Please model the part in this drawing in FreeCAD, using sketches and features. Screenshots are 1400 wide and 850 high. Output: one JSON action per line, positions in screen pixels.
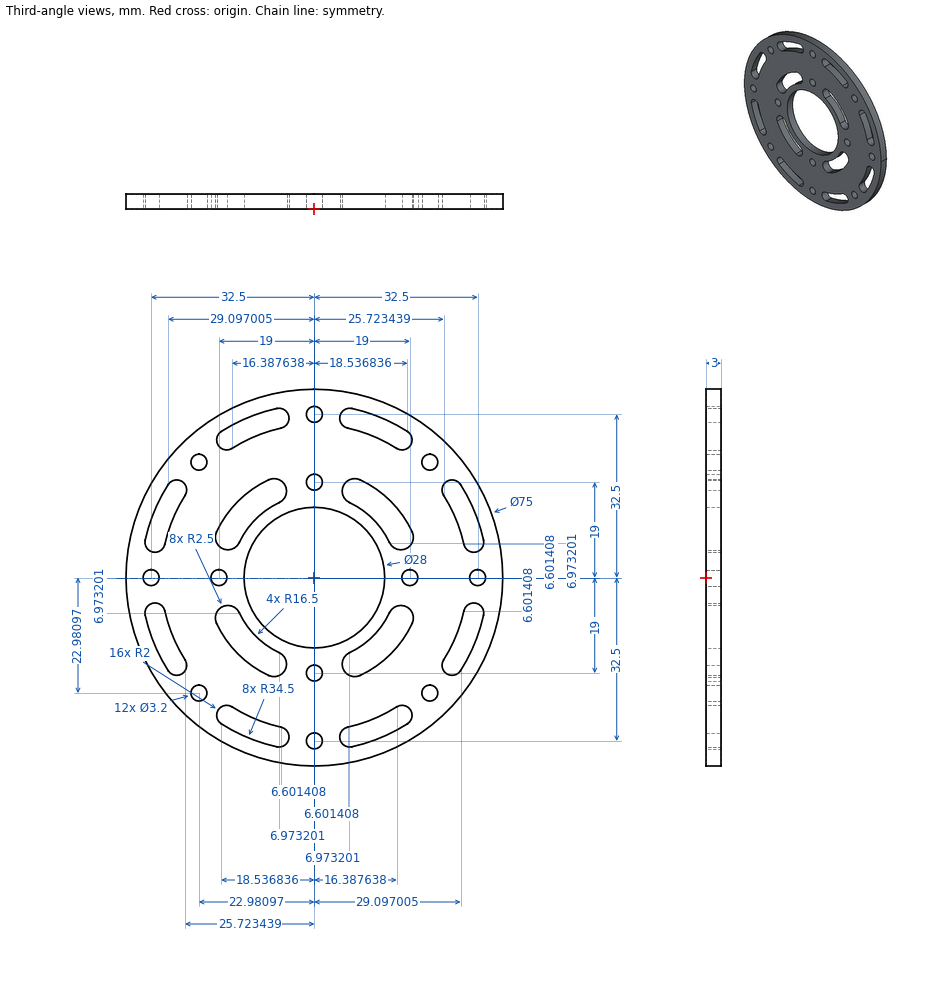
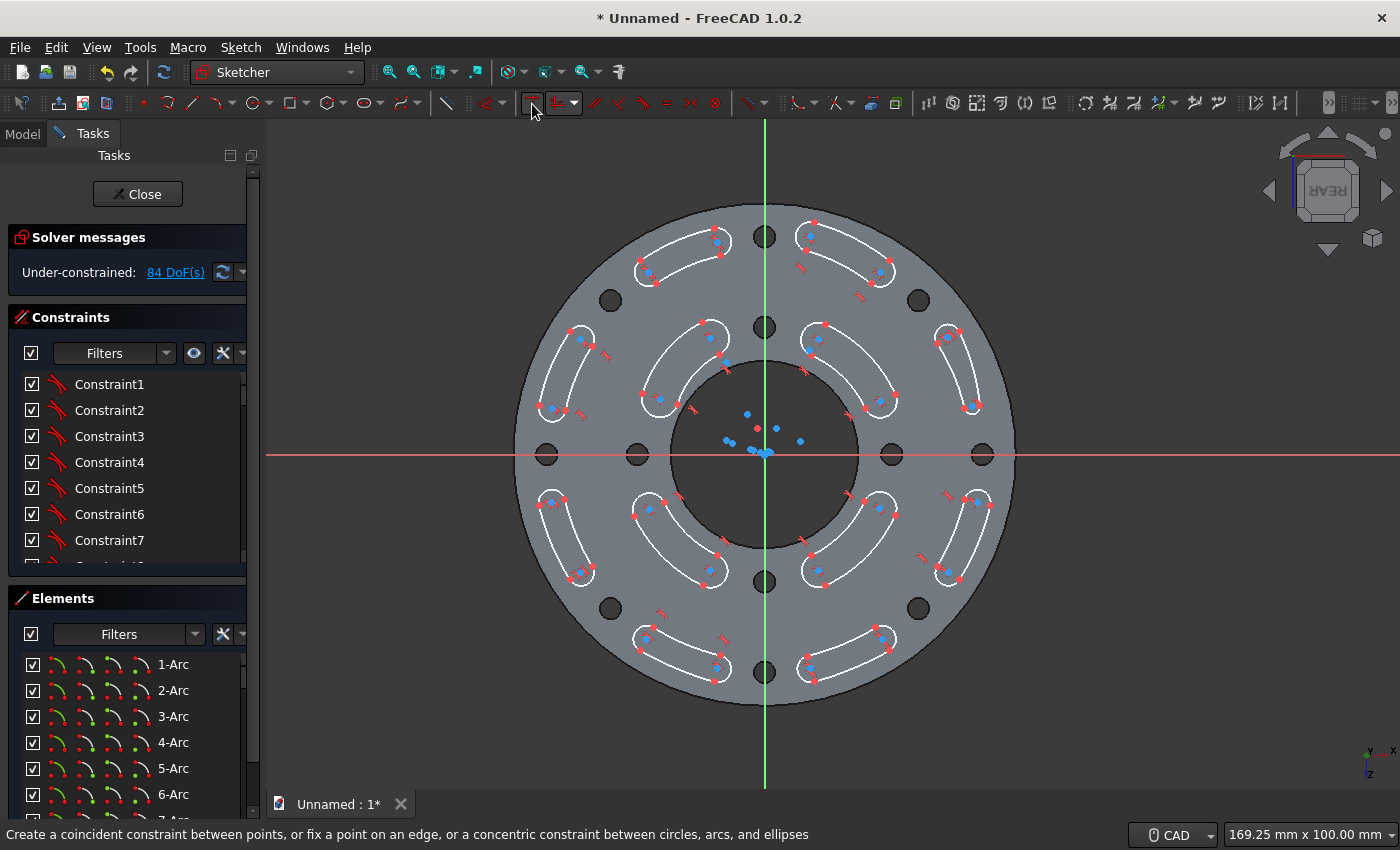
{"action": "left_click", "coordinate": [691, 235]}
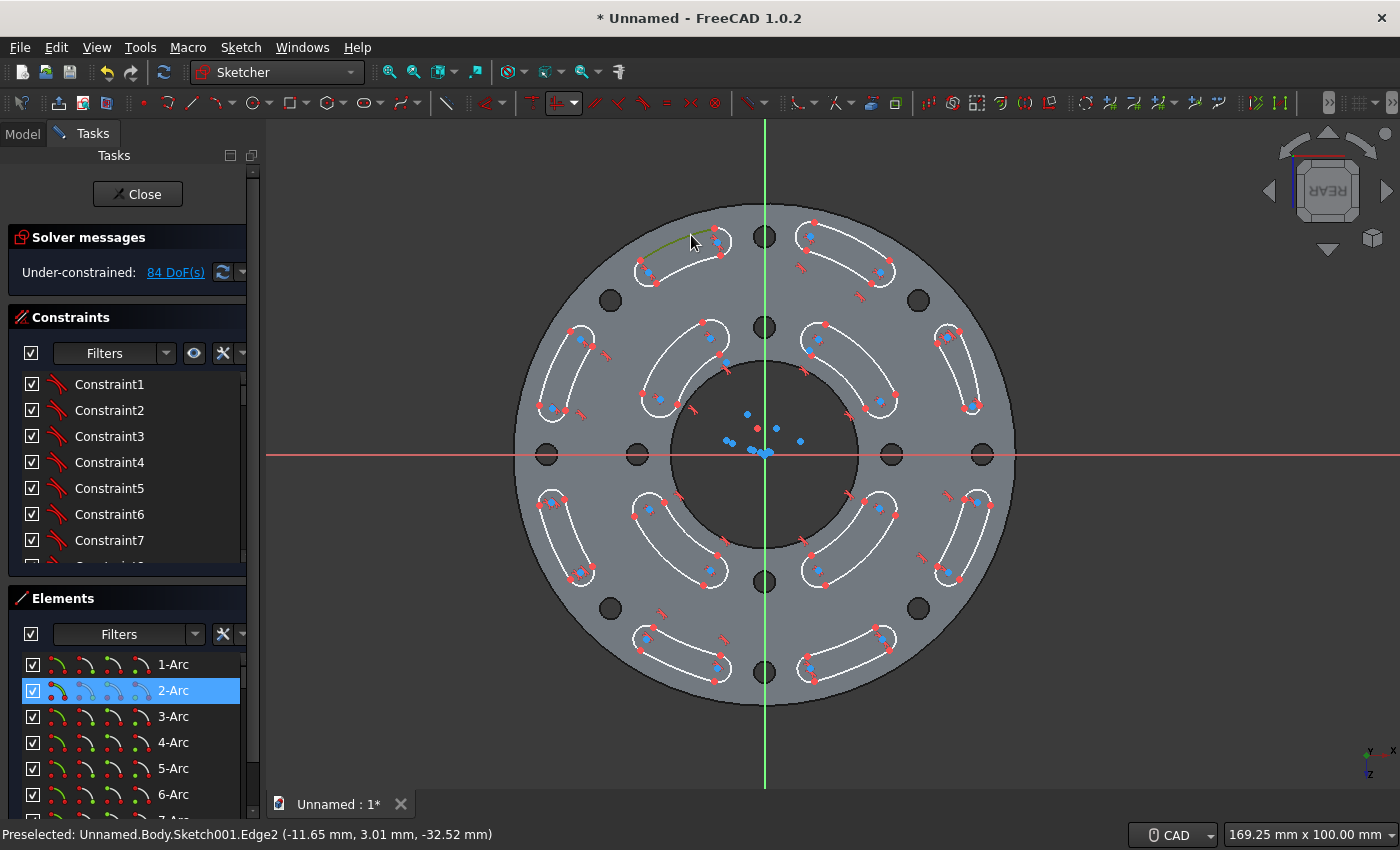
{"action": "left_click", "coordinate": [959, 388]}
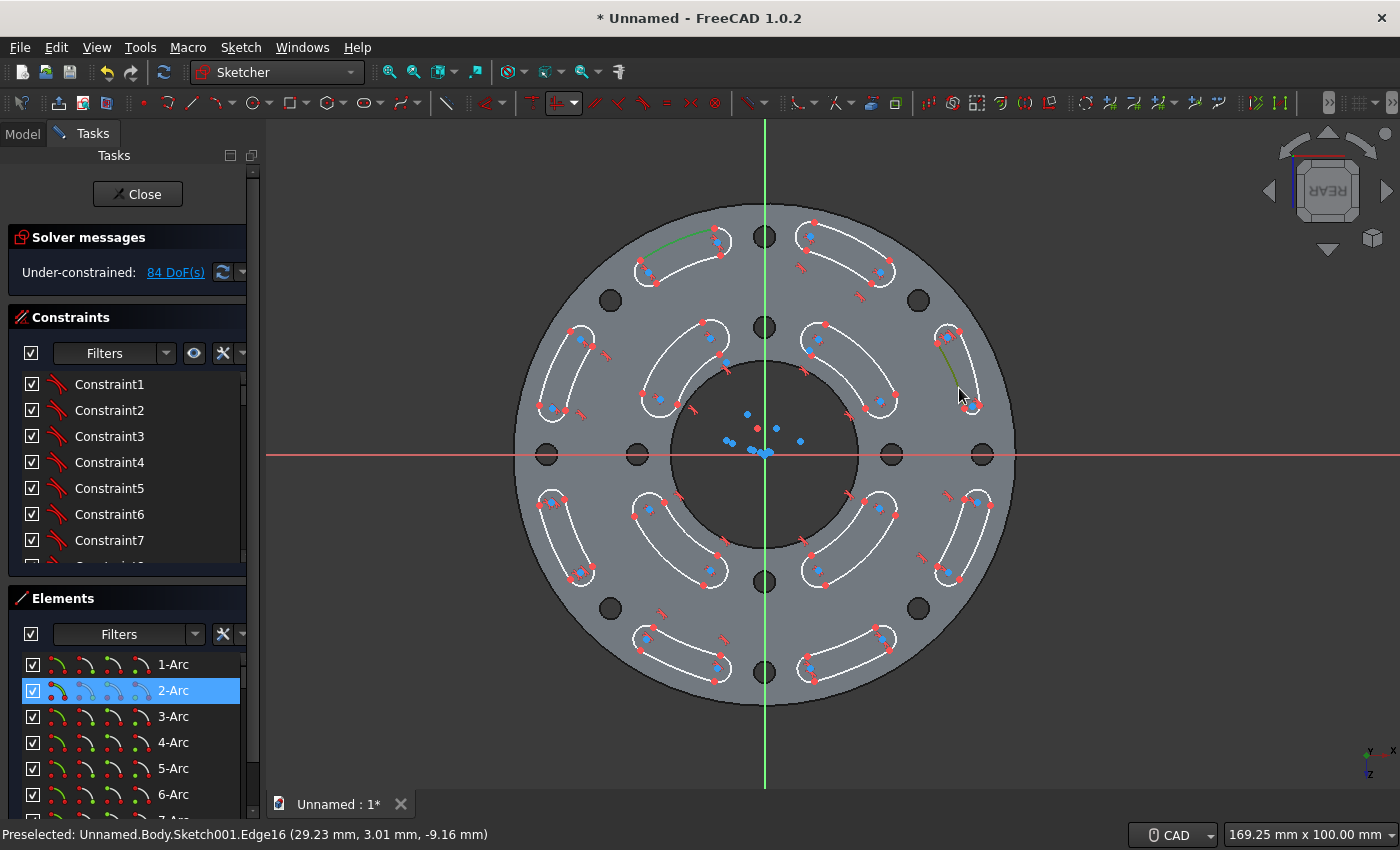
{"action": "left_click", "coordinate": [532, 104]}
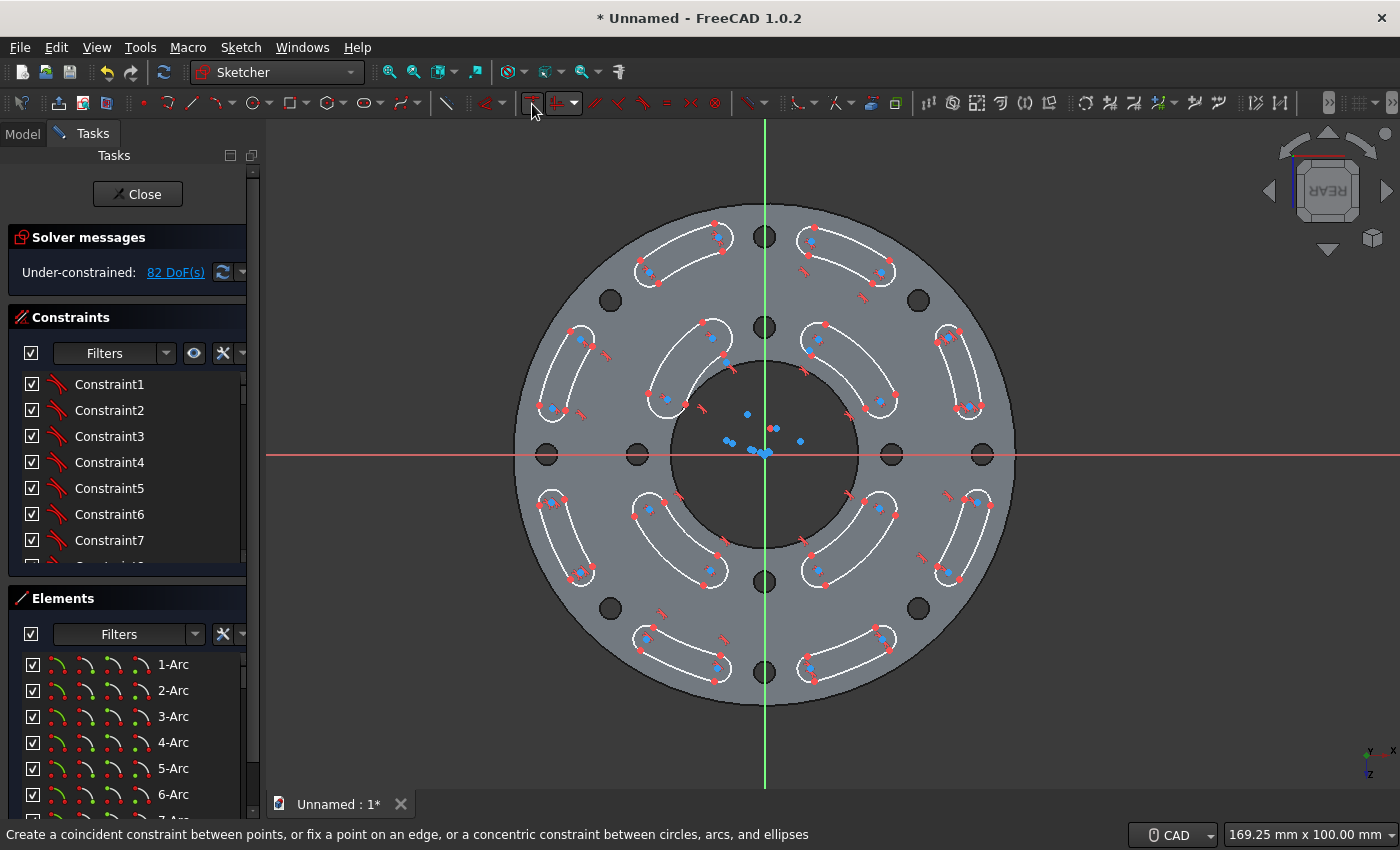
{"action": "left_click", "coordinate": [691, 232]}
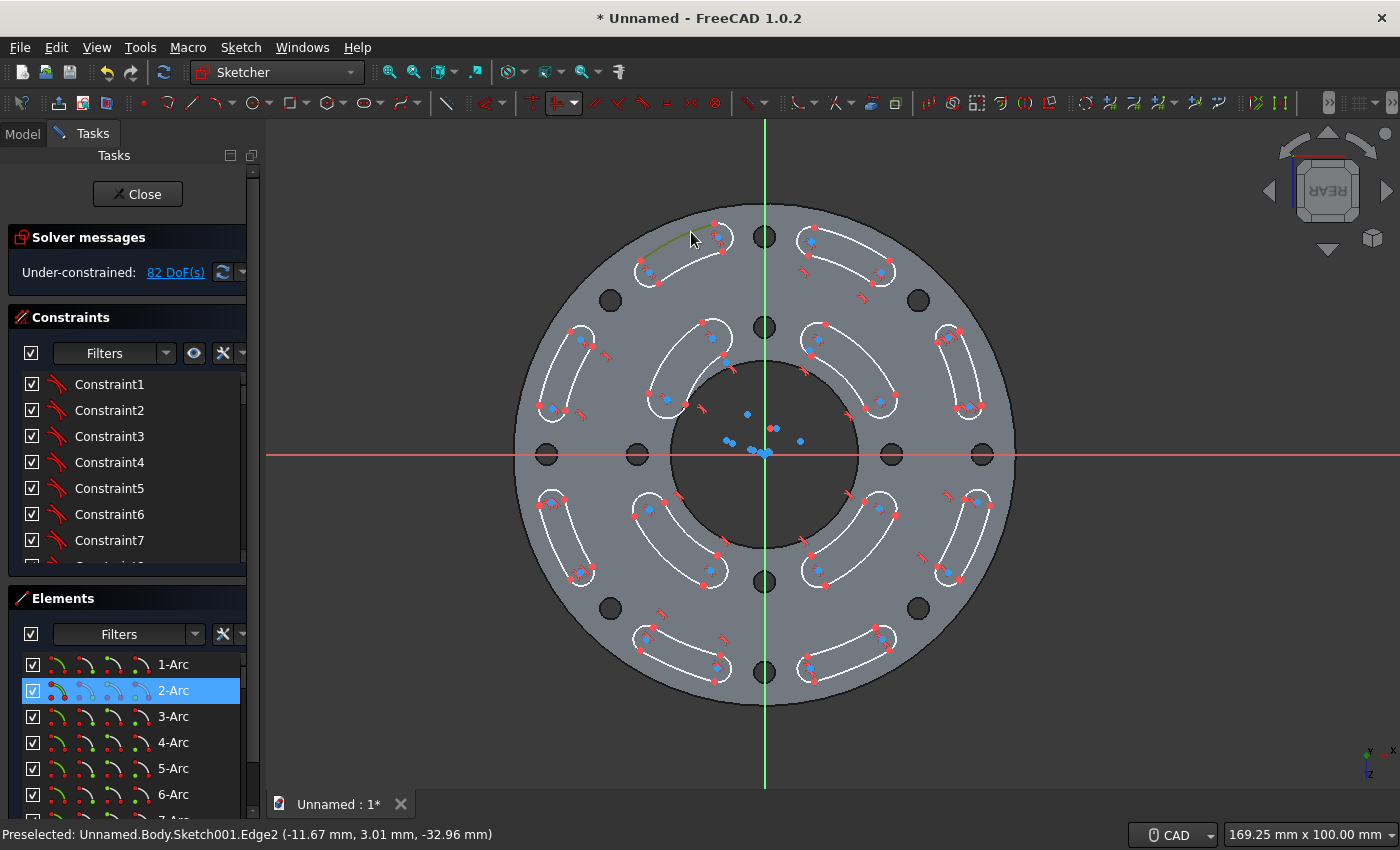
{"action": "left_click", "coordinate": [948, 547]}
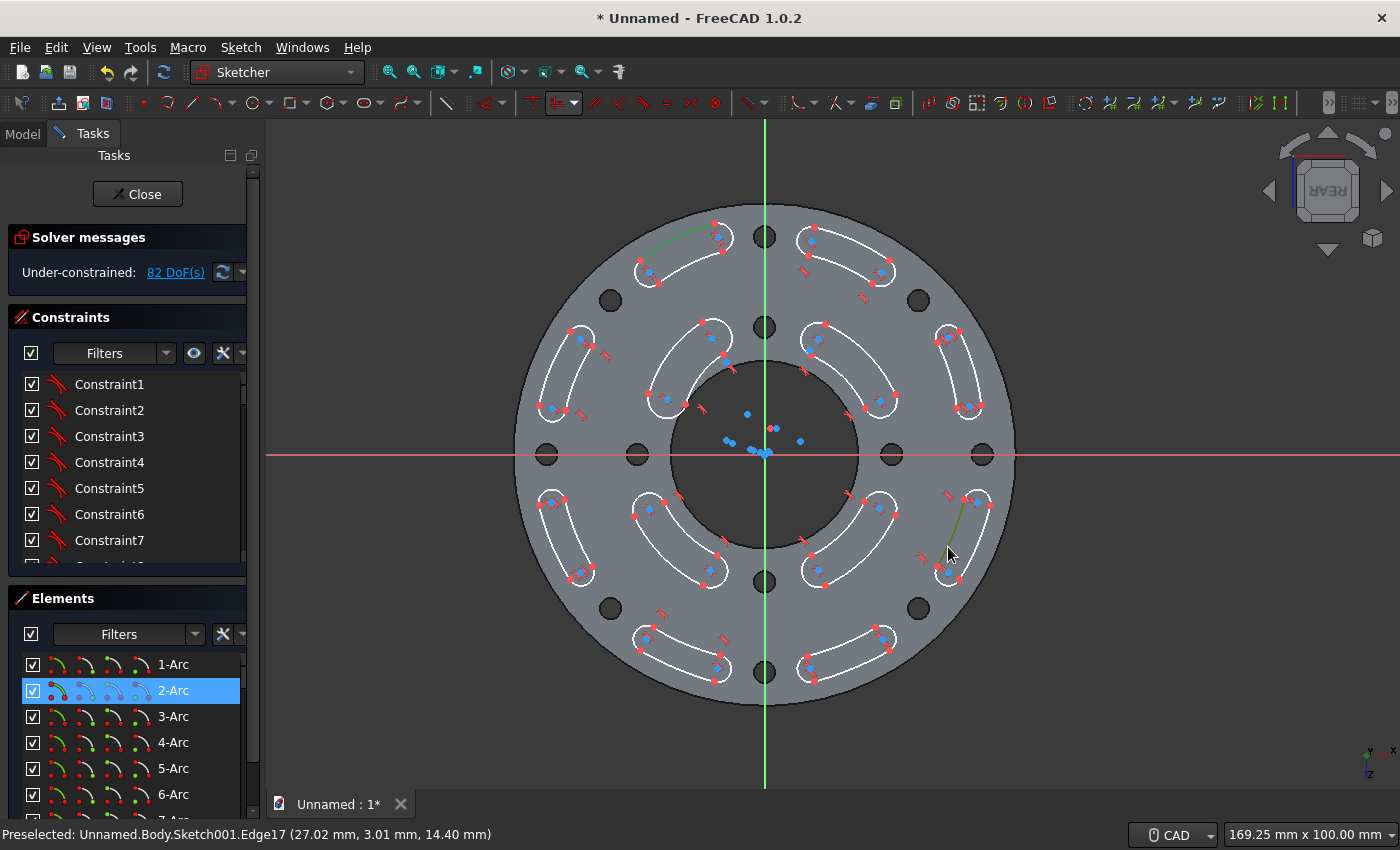
{"action": "left_click", "coordinate": [532, 104]}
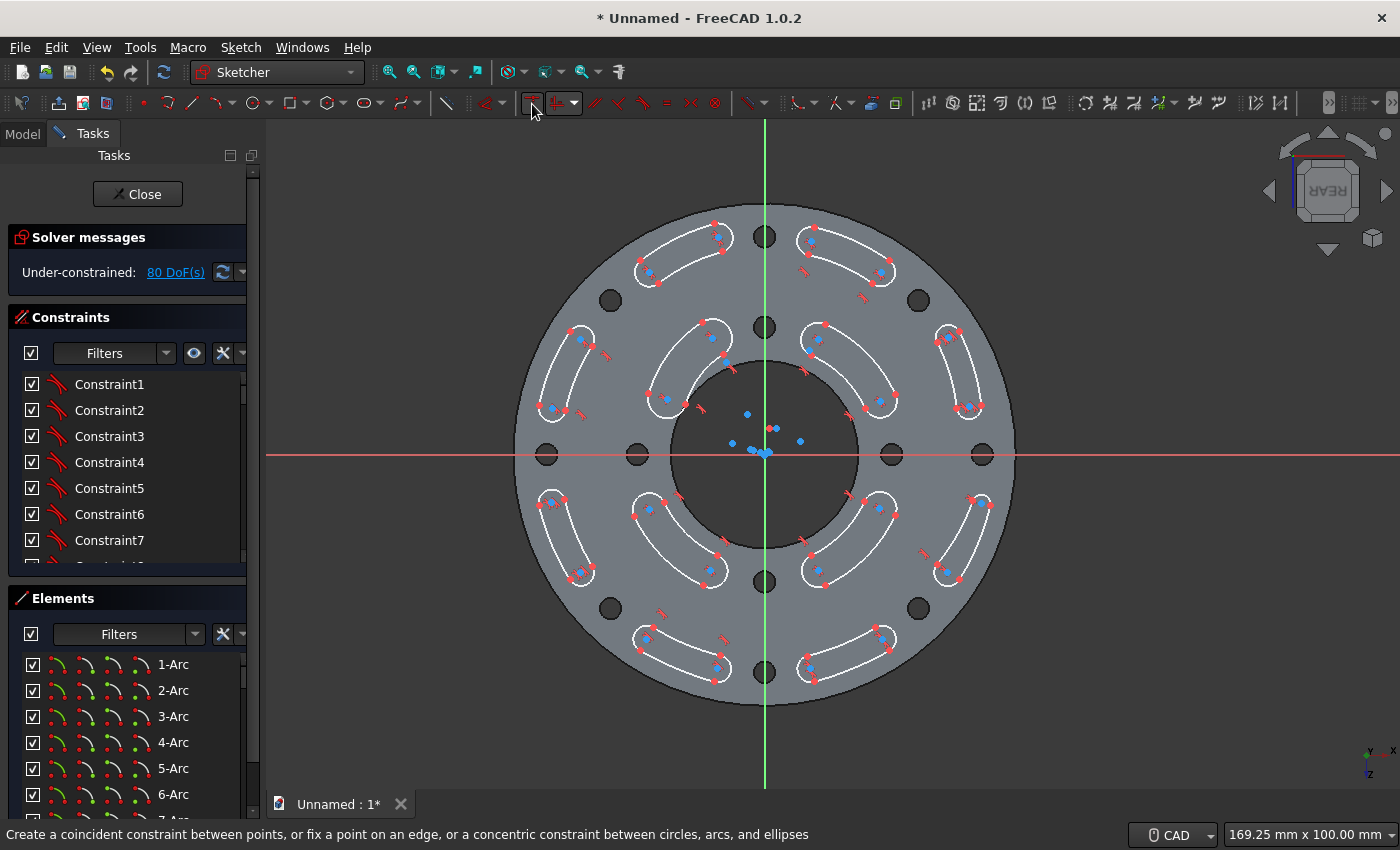
{"action": "left_click", "coordinate": [691, 232]}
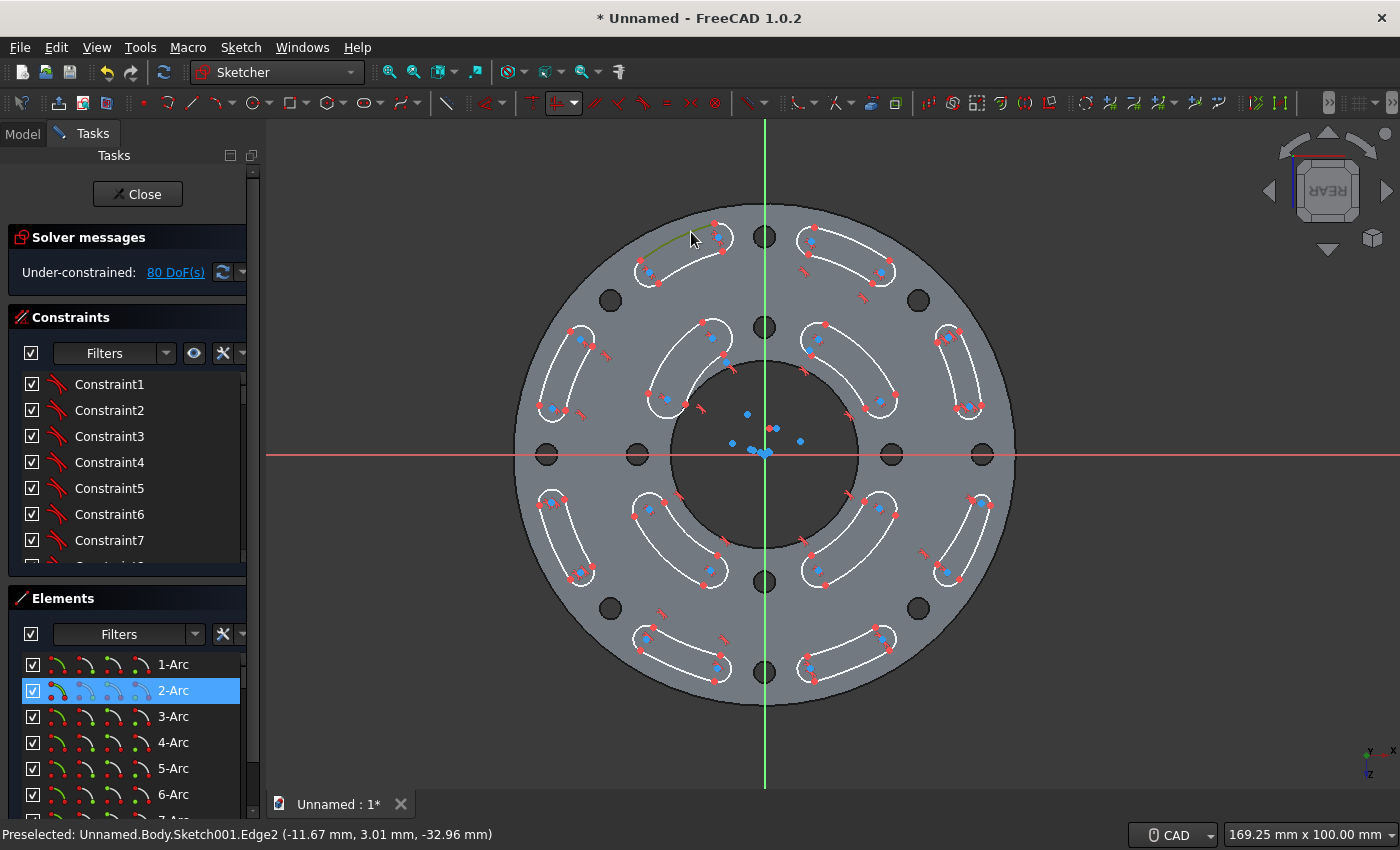
{"action": "left_click", "coordinate": [971, 559]}